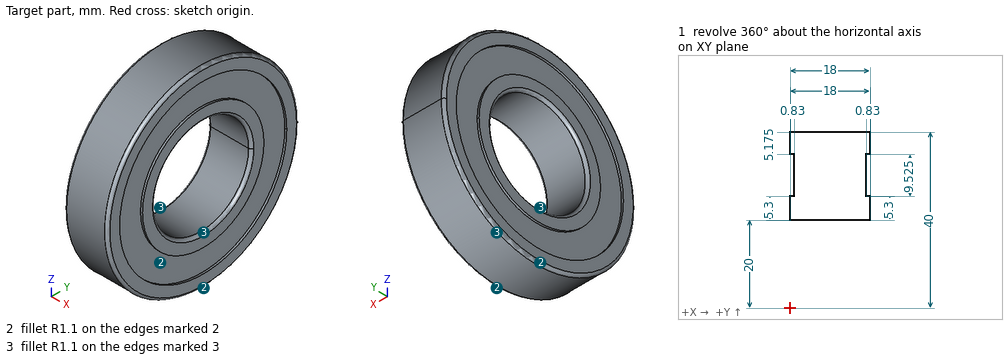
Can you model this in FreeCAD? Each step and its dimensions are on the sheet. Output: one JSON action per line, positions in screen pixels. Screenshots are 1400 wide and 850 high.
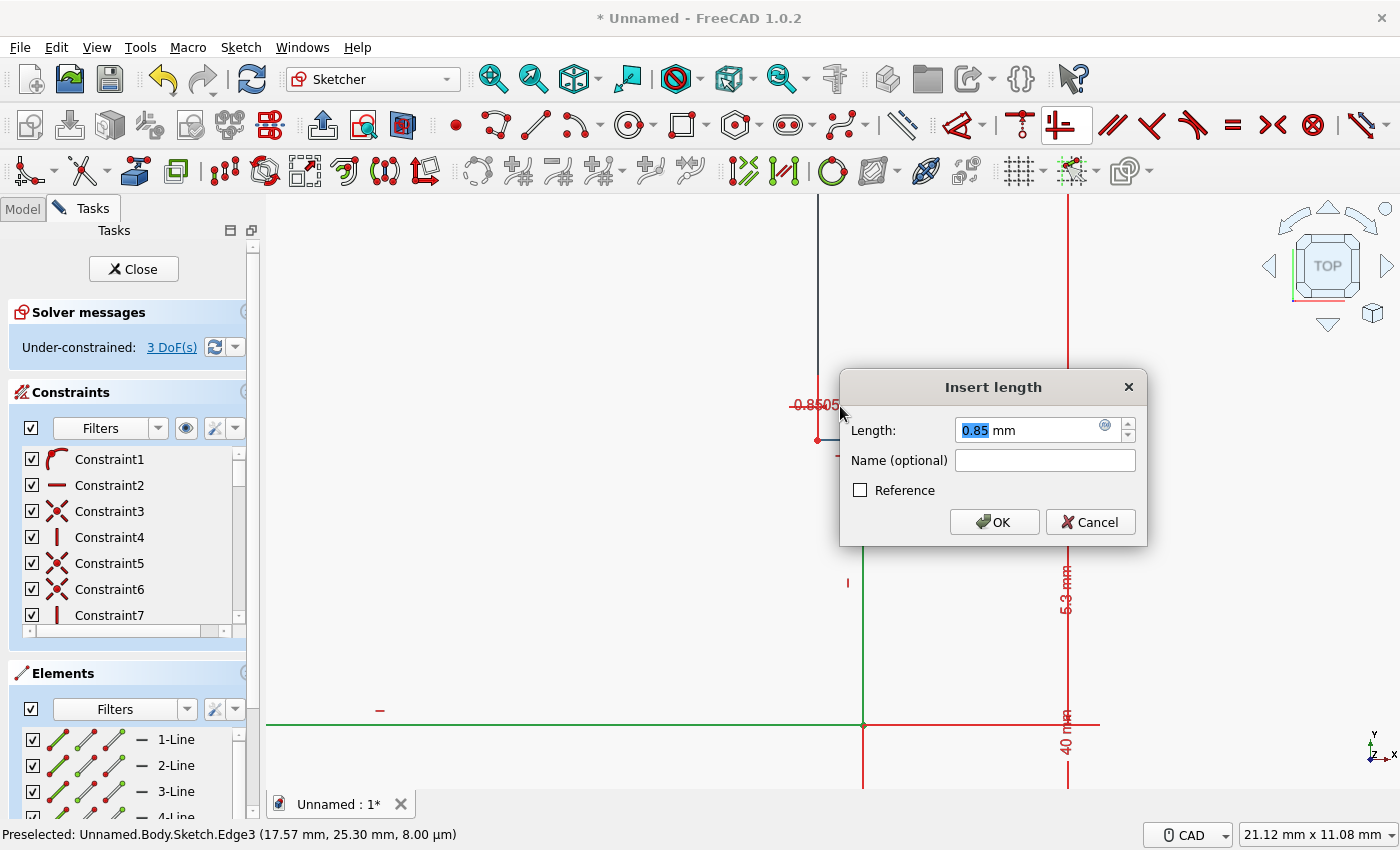
{"action": "type", "text": "0.83"}
{"action": "key", "text": "Return"}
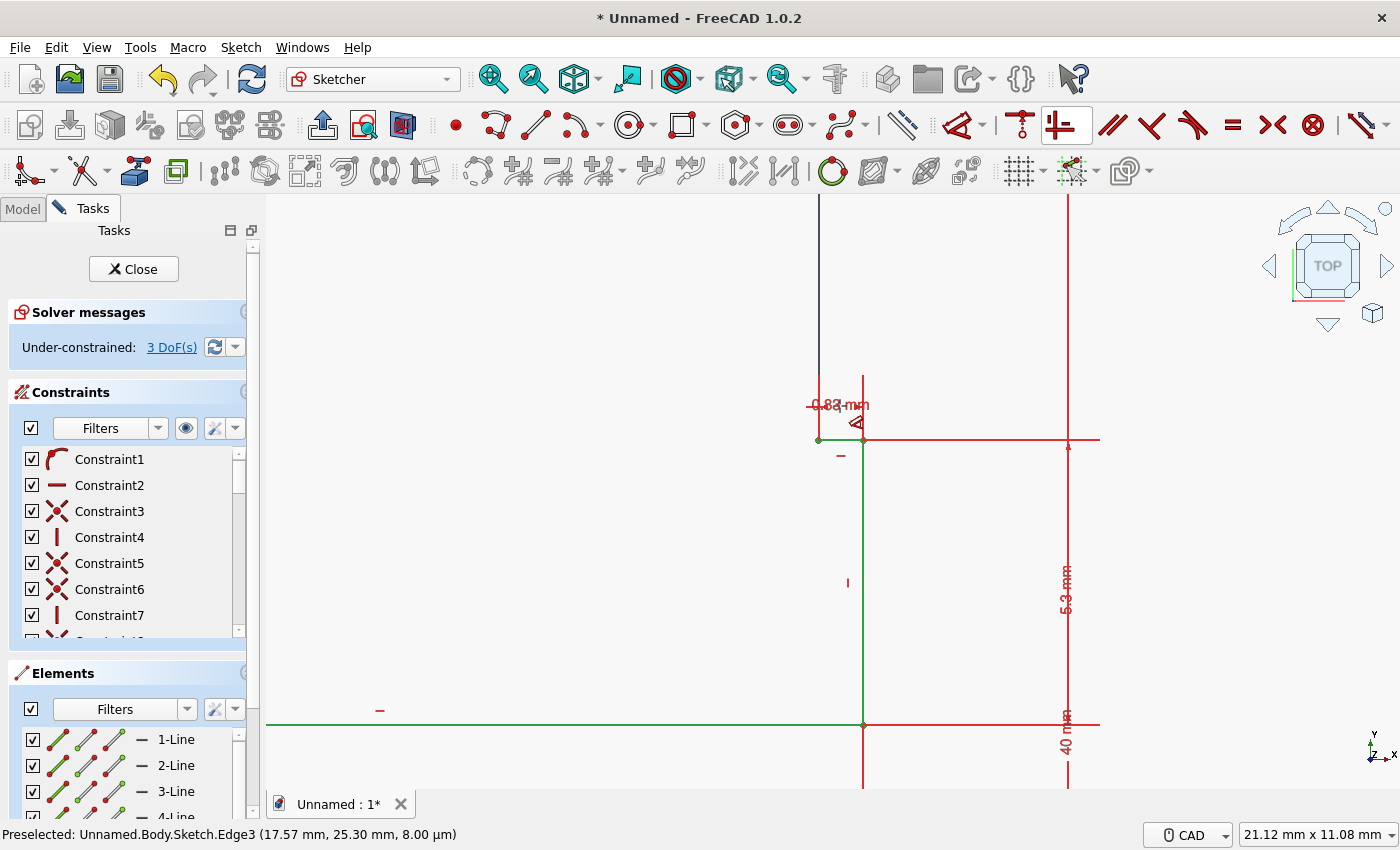
{"action": "scroll", "coordinate": [841, 445], "scroll_direction": "down", "scroll_amount": 9}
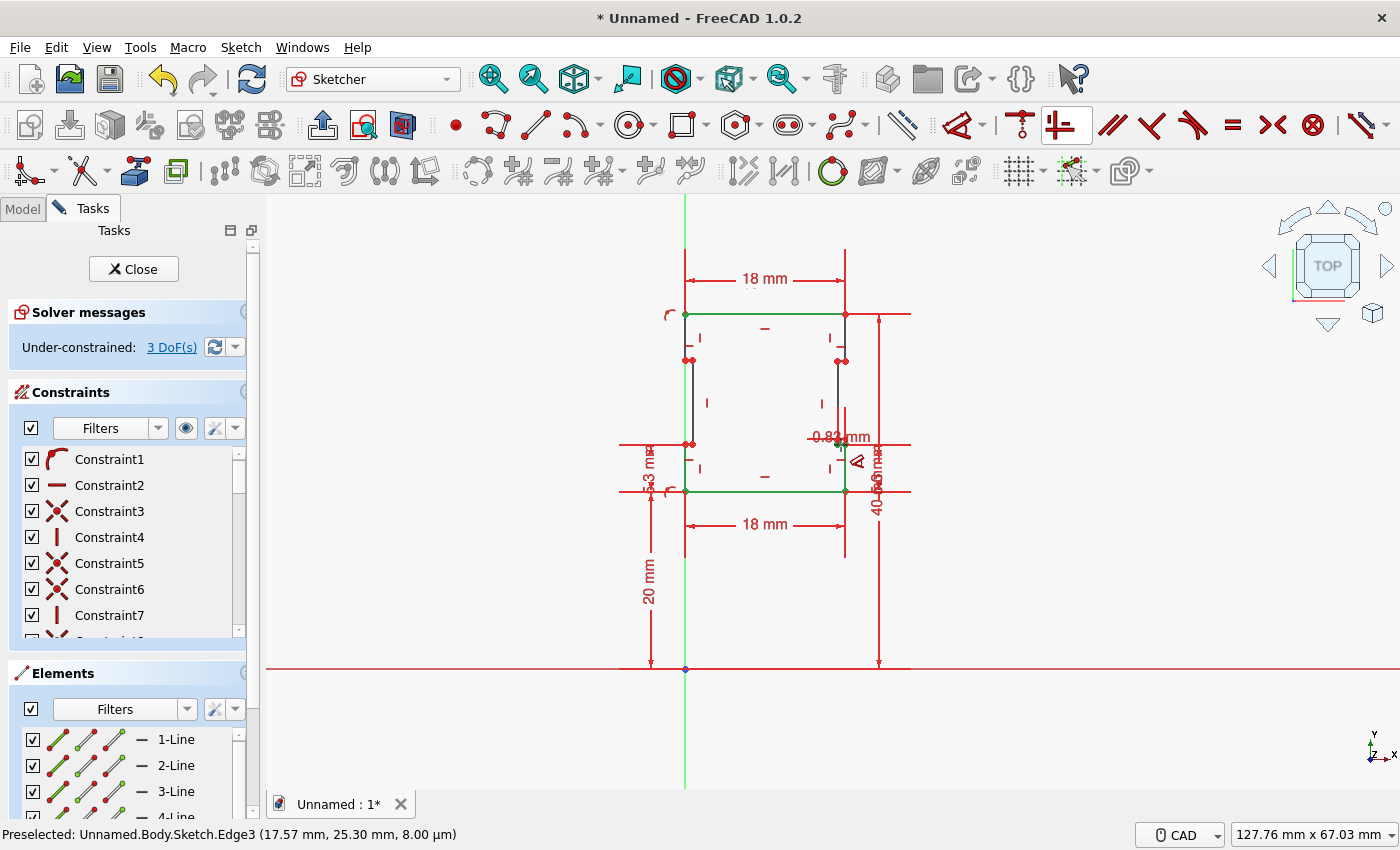
{"action": "scroll", "coordinate": [688, 361], "scroll_direction": "up", "scroll_amount": 10}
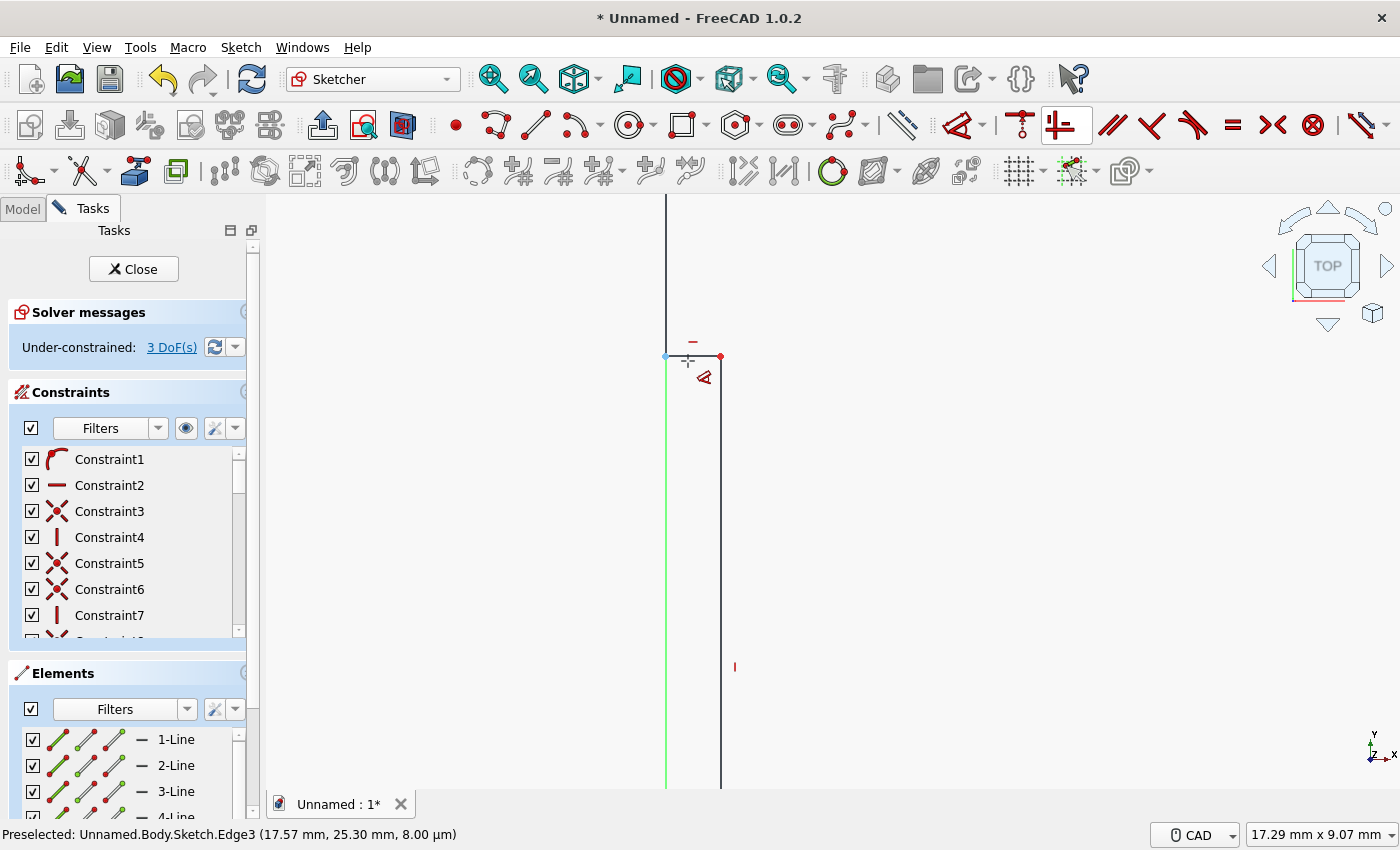
{"action": "left_click", "coordinate": [682, 356]}
{"action": "left_click", "coordinate": [693, 322]}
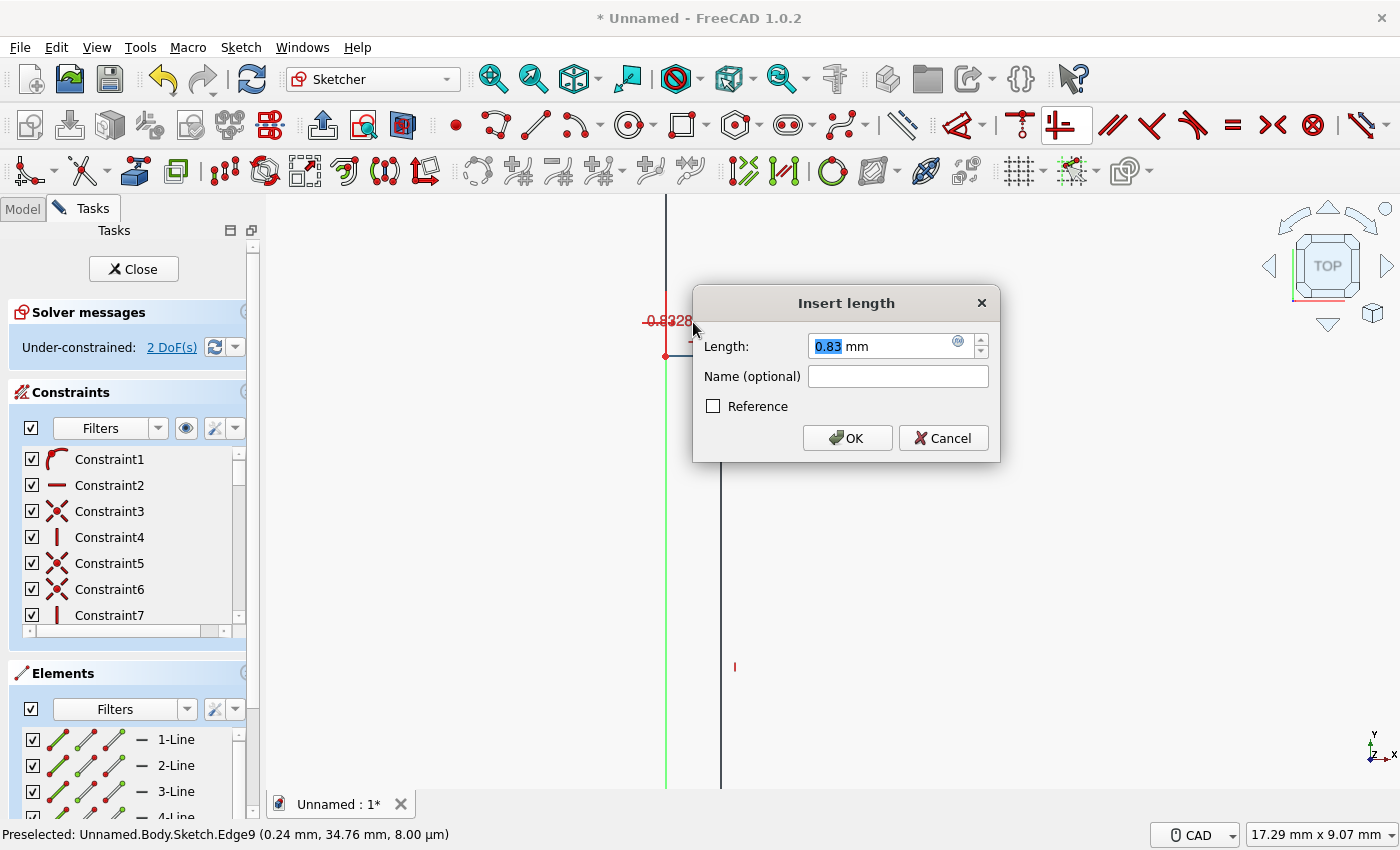
{"action": "type", "text": "0.83"}
{"action": "key", "text": "Return"}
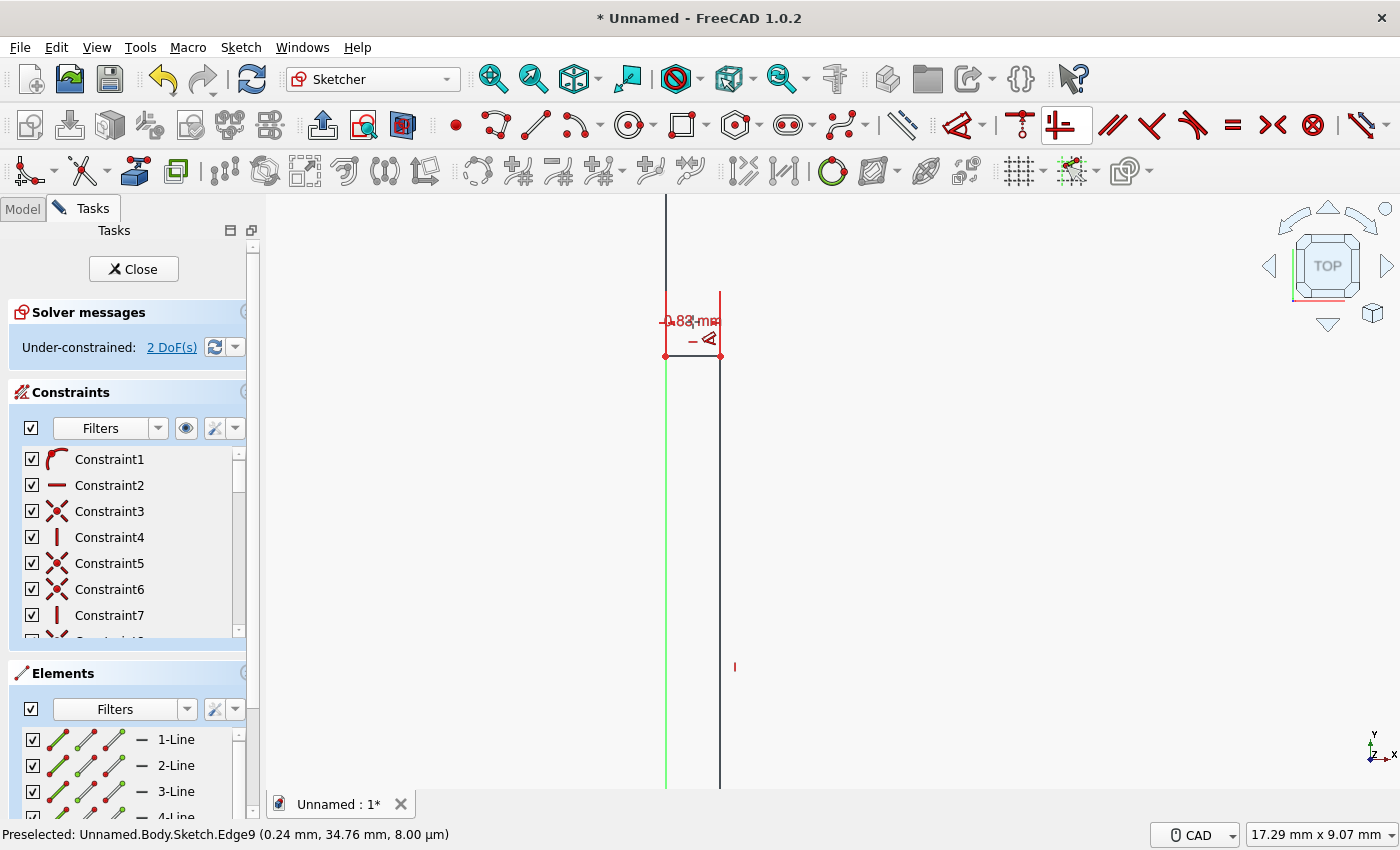
{"action": "scroll", "coordinate": [688, 361], "scroll_direction": "down", "scroll_amount": 10}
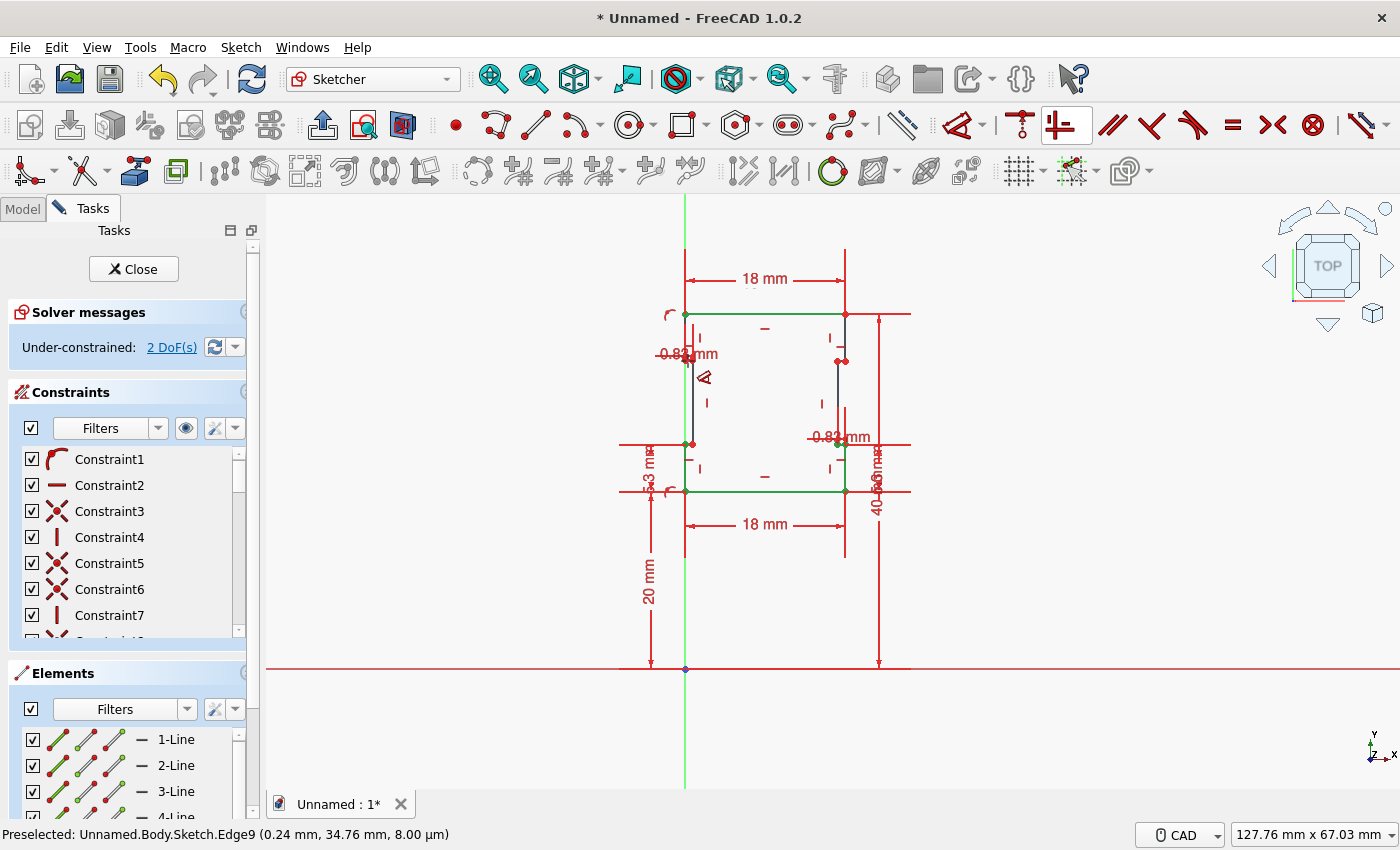
{"action": "left_click", "coordinate": [838, 420]}
{"action": "left_click", "coordinate": [872, 403]}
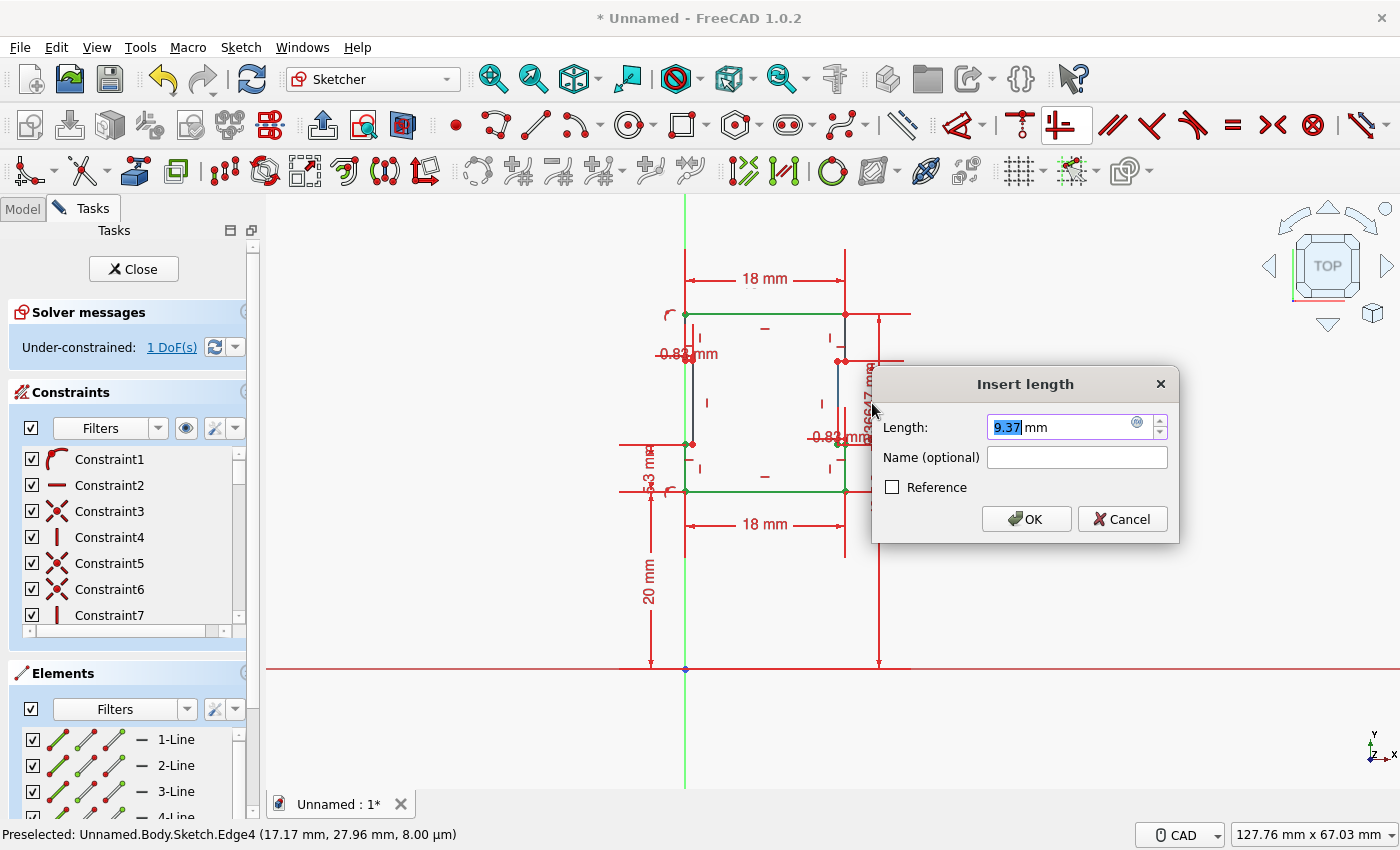
{"action": "type", "text": "9.525"}
{"action": "key", "text": "Return"}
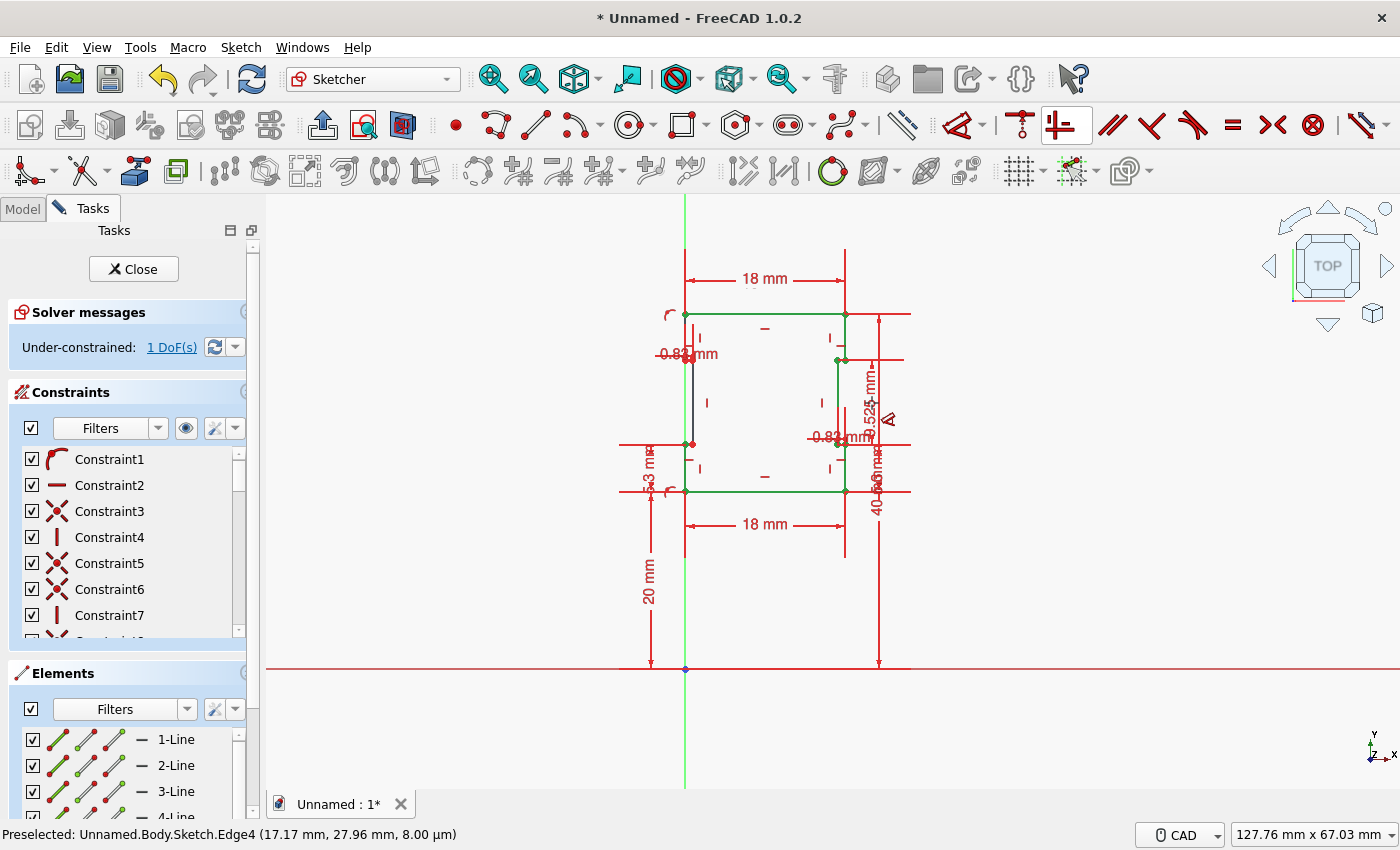
{"action": "left_click", "coordinate": [685, 328]}
{"action": "left_click", "coordinate": [651, 327]}